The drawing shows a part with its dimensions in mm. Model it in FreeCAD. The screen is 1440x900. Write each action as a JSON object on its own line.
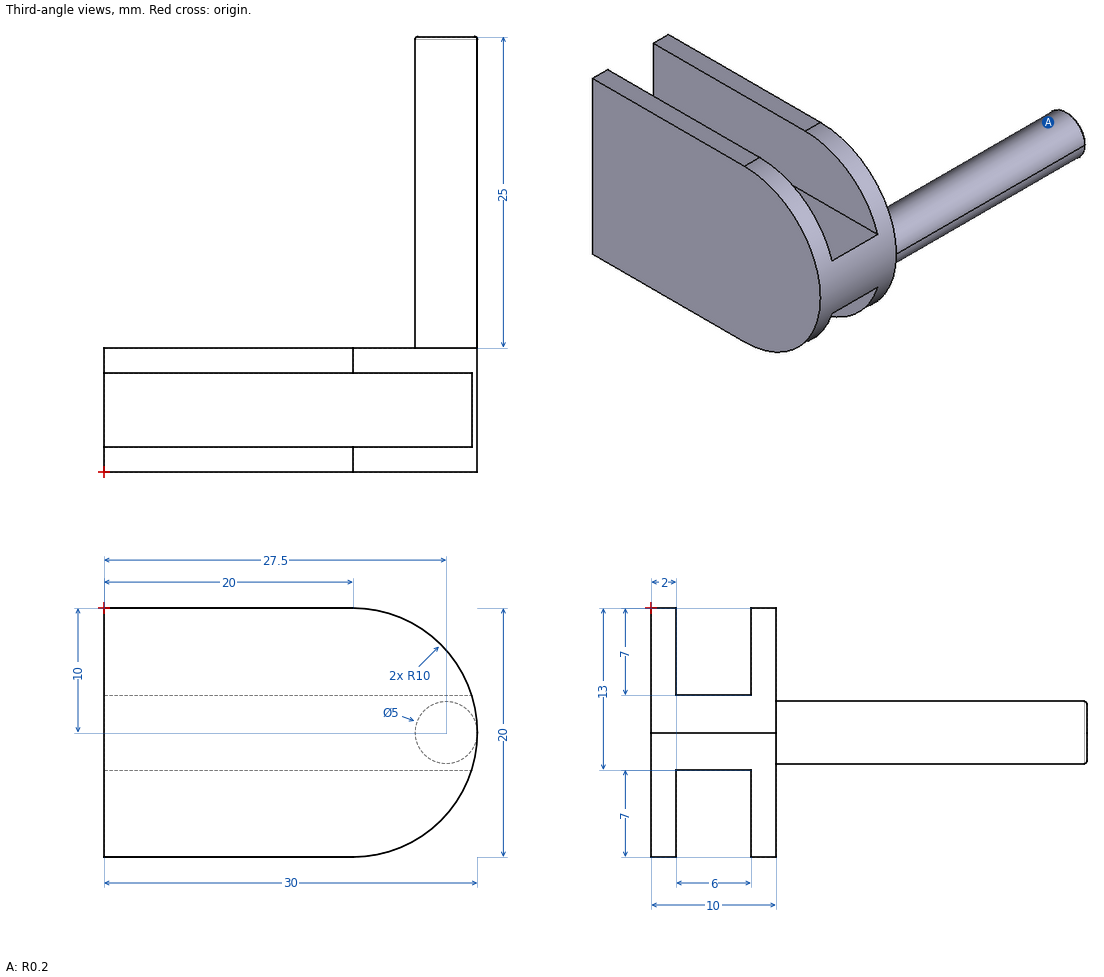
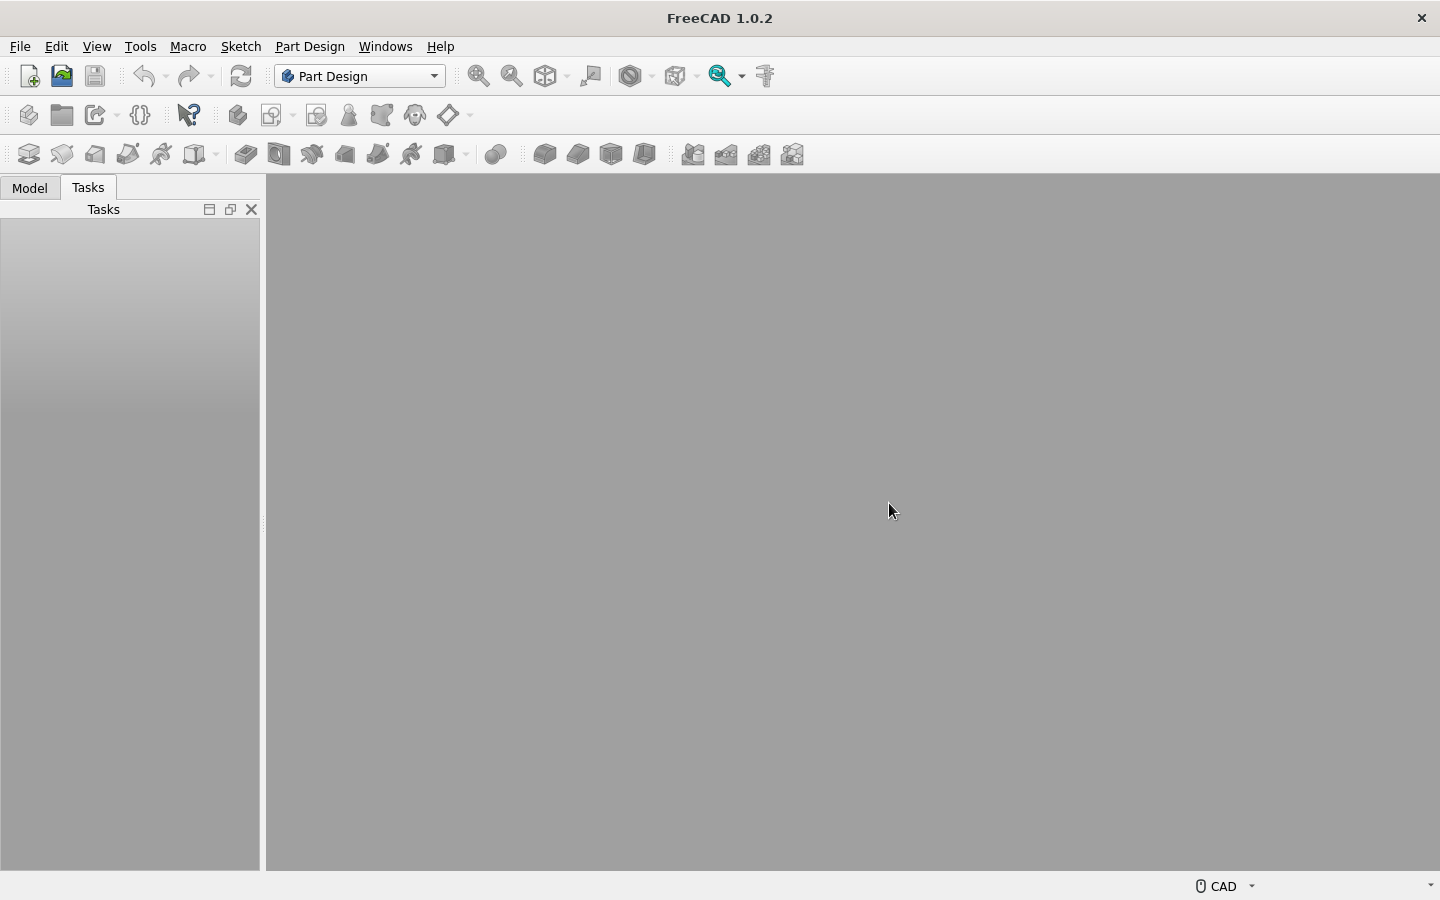
{"action": "left_click", "coordinate": [29, 76]}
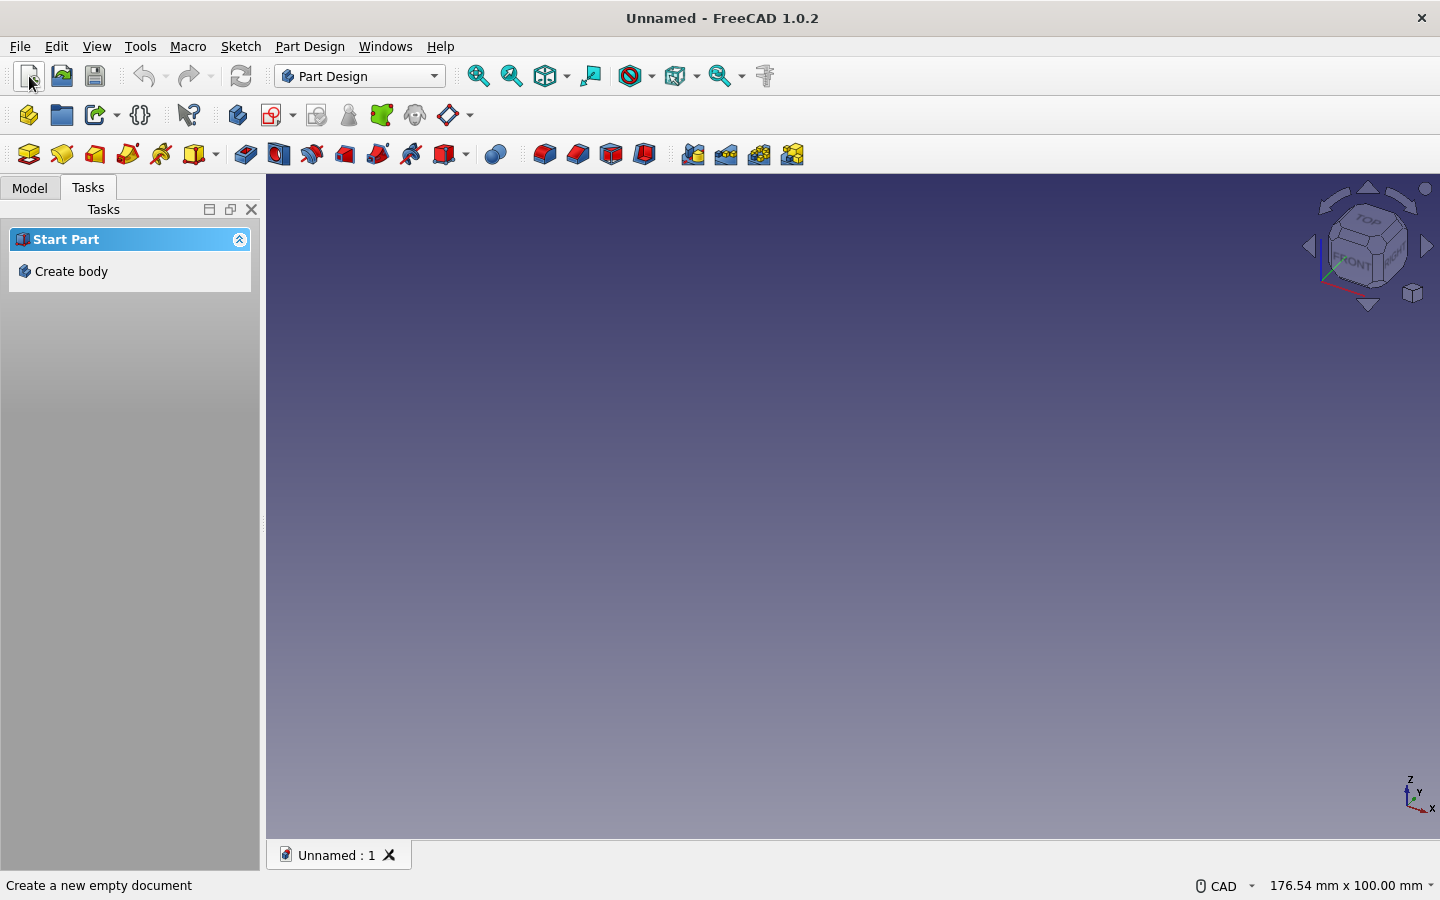
{"action": "left_click", "coordinate": [270, 116]}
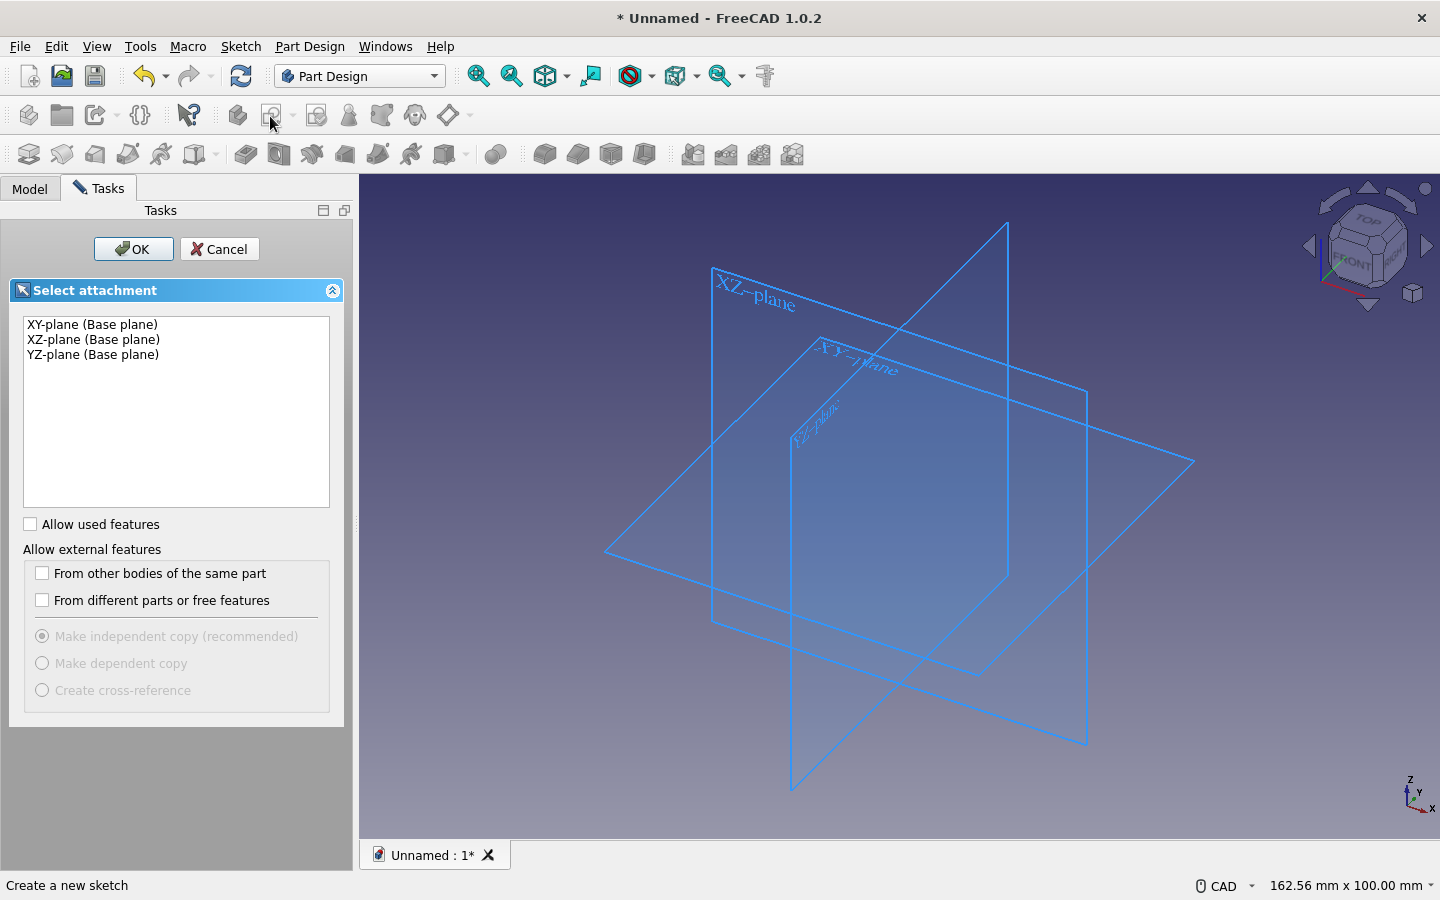
{"action": "left_click", "coordinate": [84, 340]}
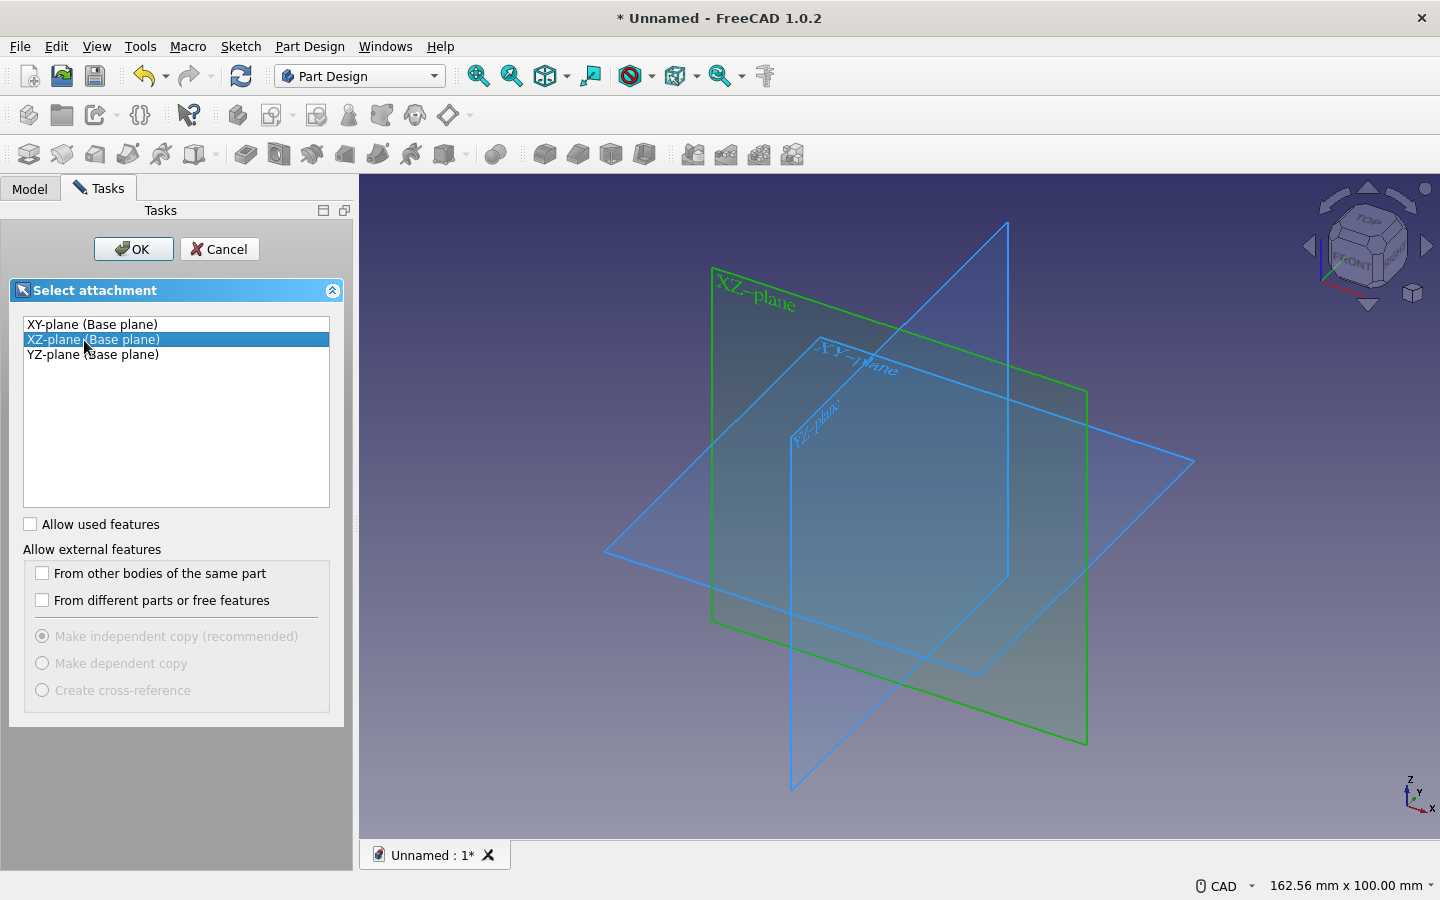
{"action": "left_click", "coordinate": [134, 249]}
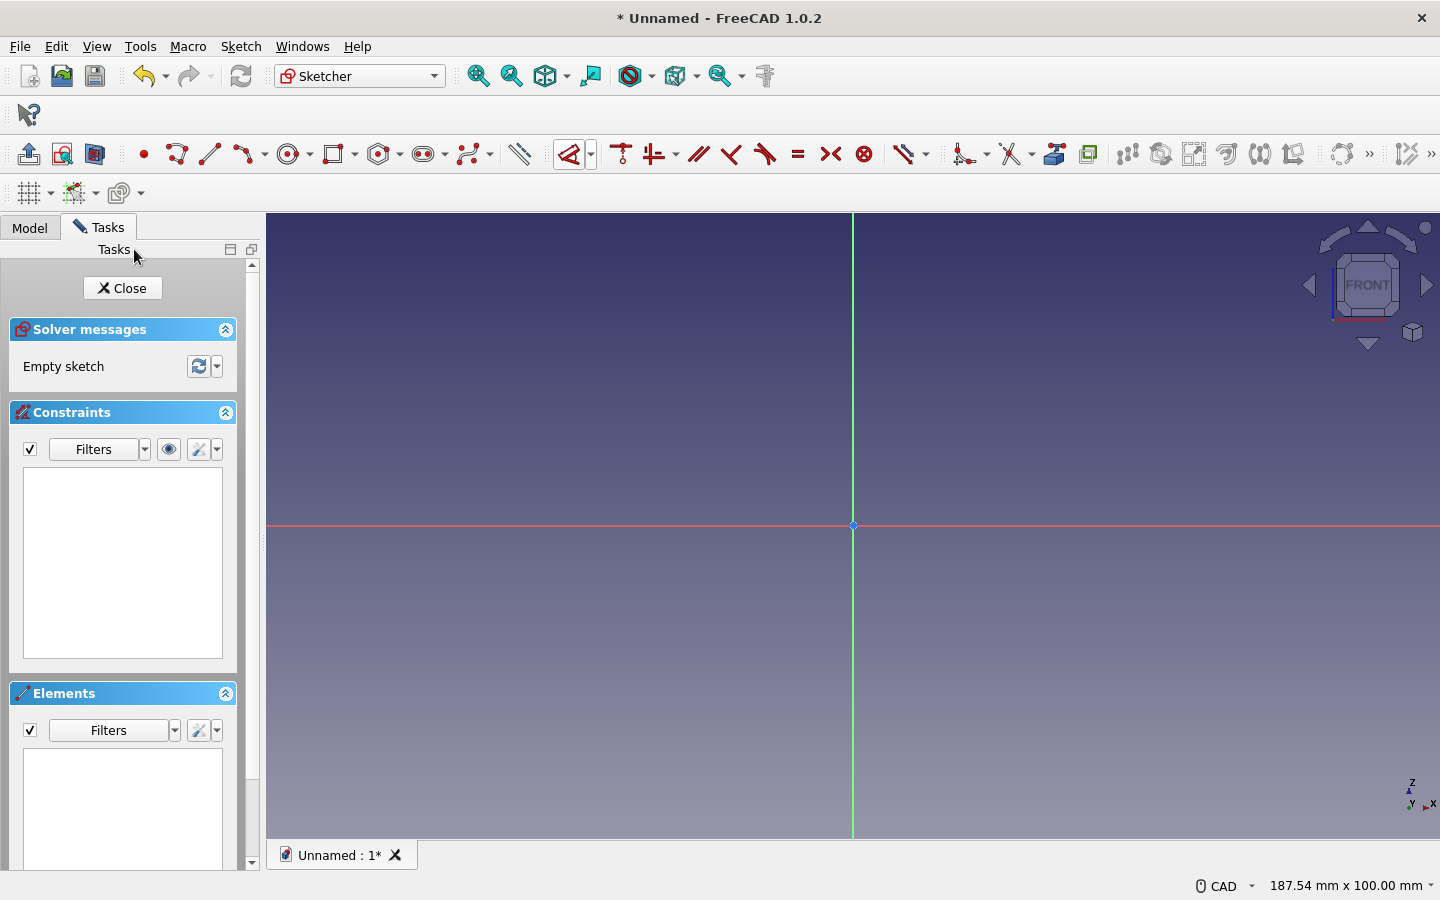
{"action": "scroll", "coordinate": [1017, 616], "scroll_direction": "up", "scroll_amount": 6}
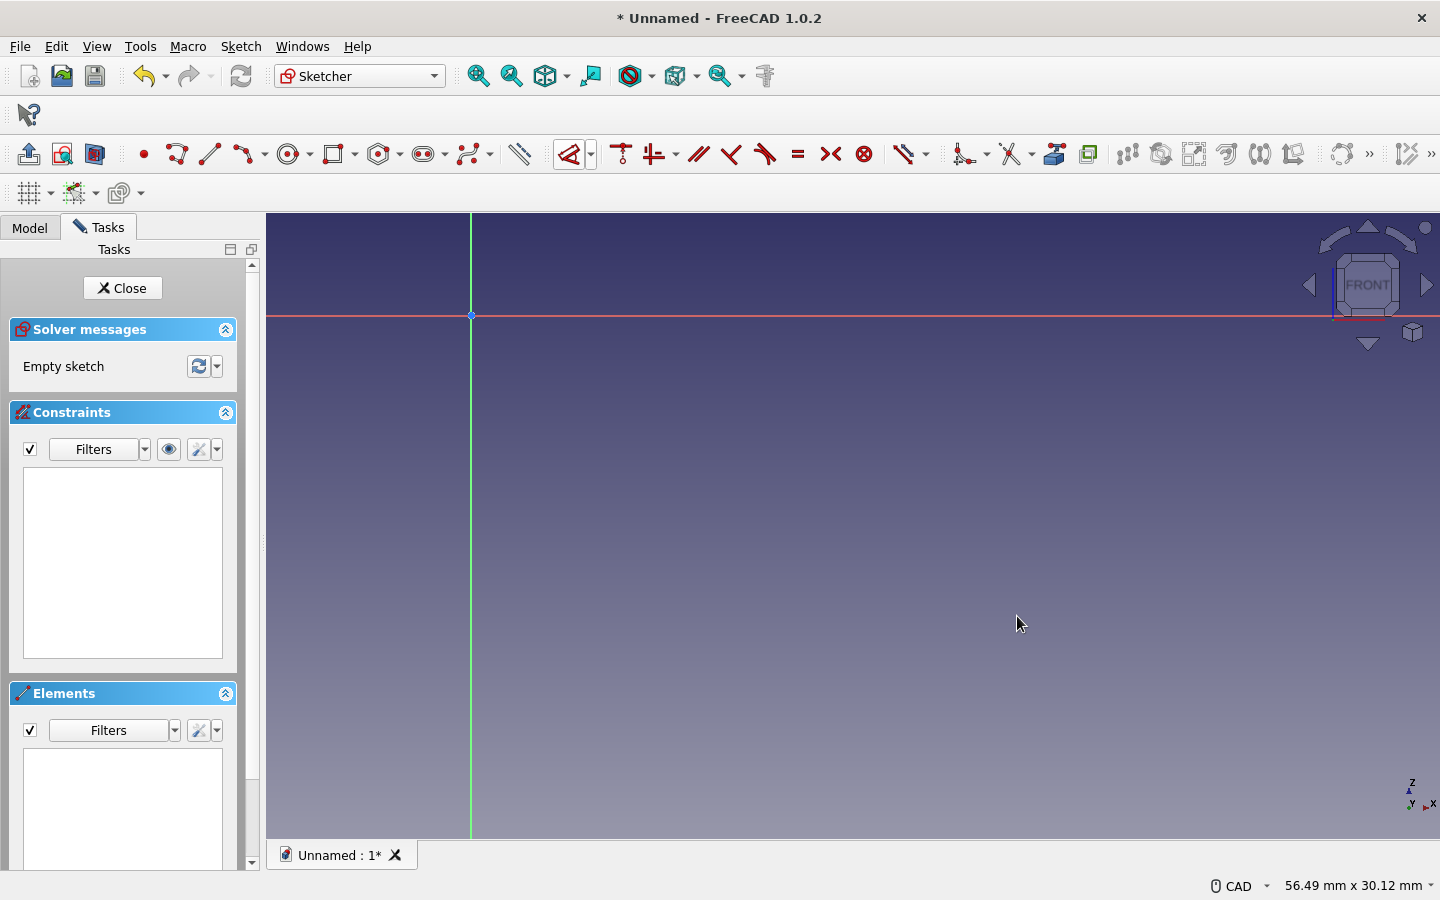
{"action": "left_click", "coordinate": [332, 154]}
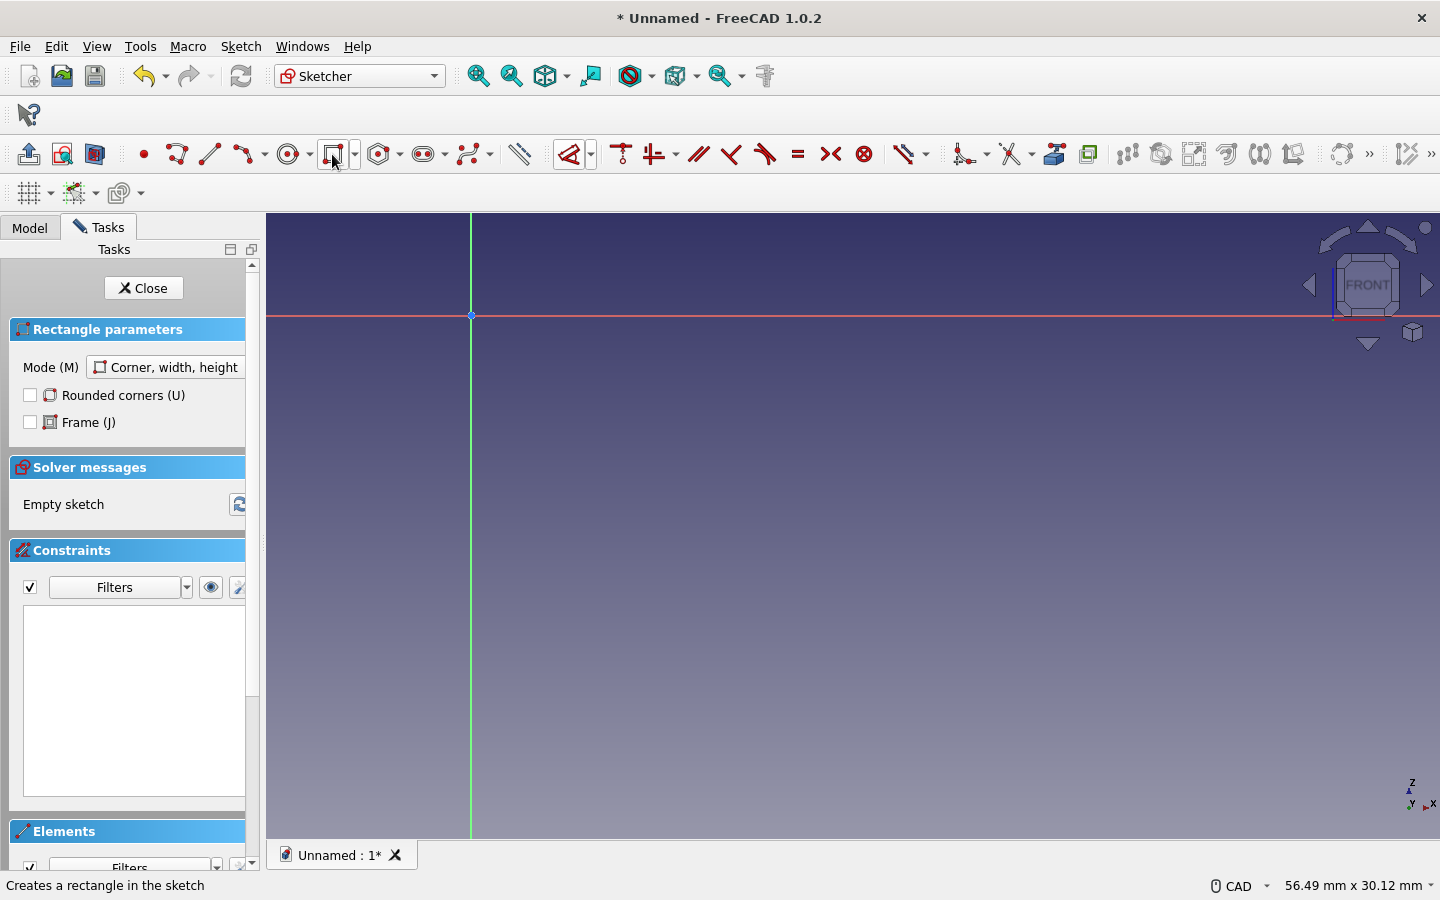
{"action": "left_click", "coordinate": [471, 316]}
{"action": "mouse_move", "coordinate": [1095, 731]}